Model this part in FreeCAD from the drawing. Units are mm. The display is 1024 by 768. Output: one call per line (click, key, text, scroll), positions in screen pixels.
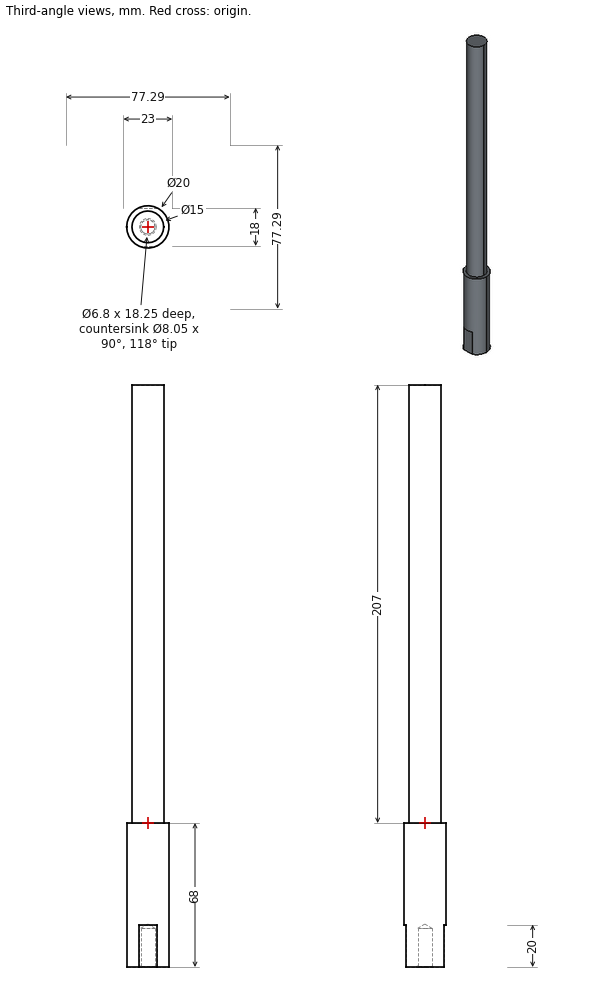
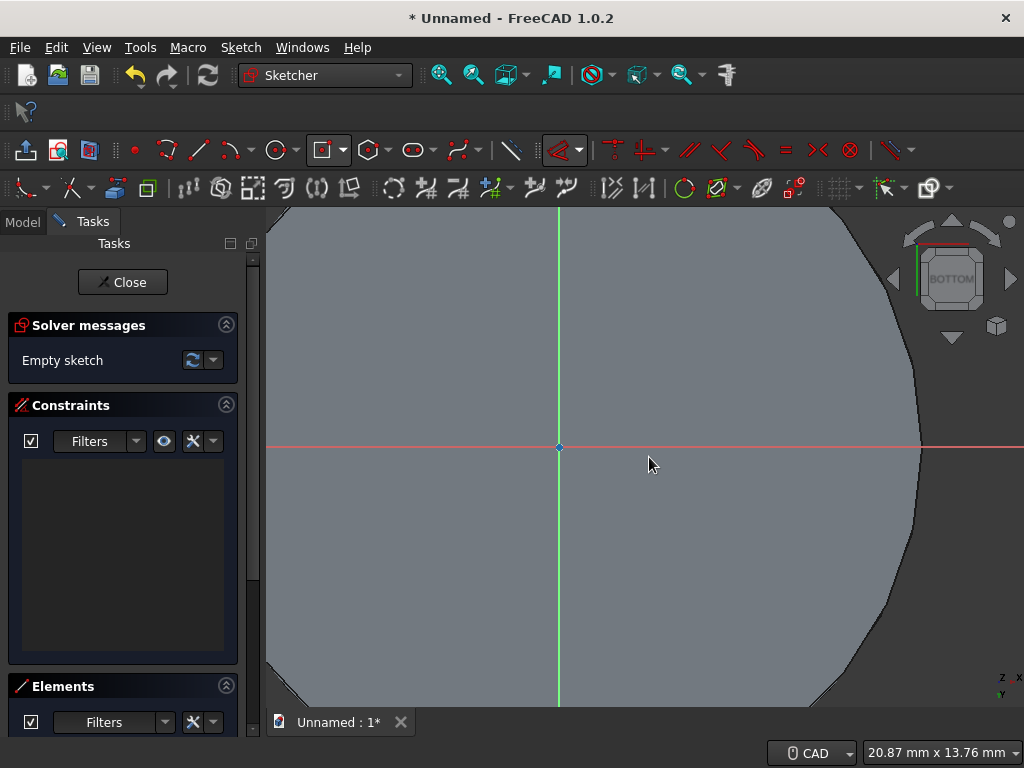
click(276, 150)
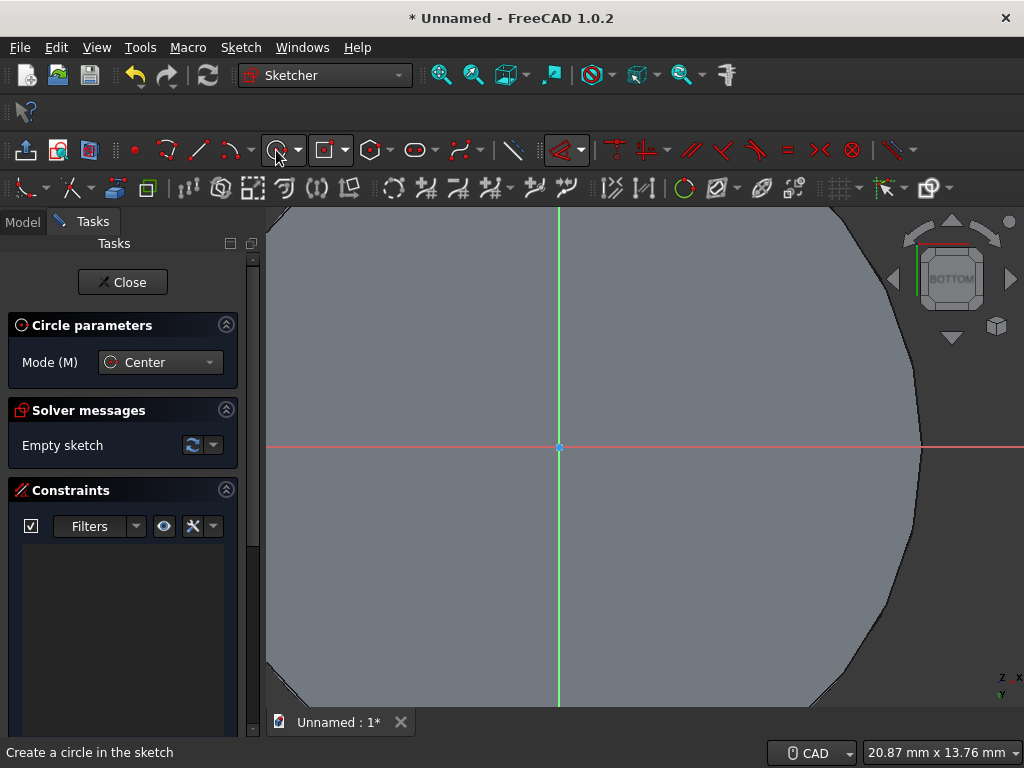
click(559, 447)
click(646, 360)
key(Escape)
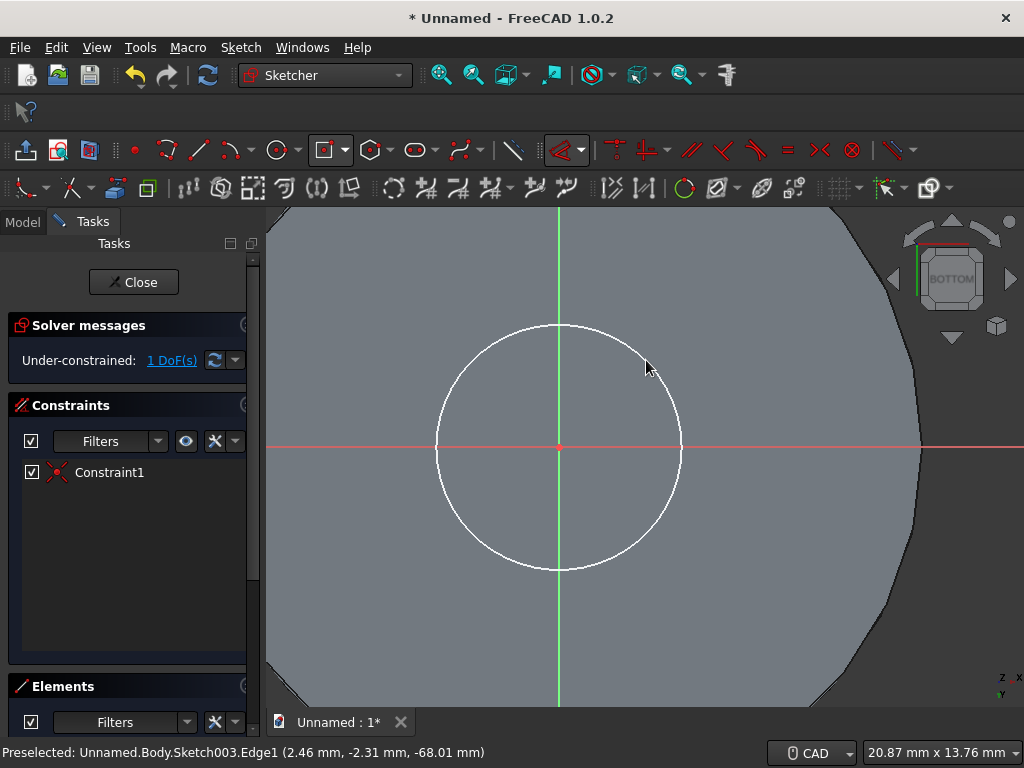
click(645, 360)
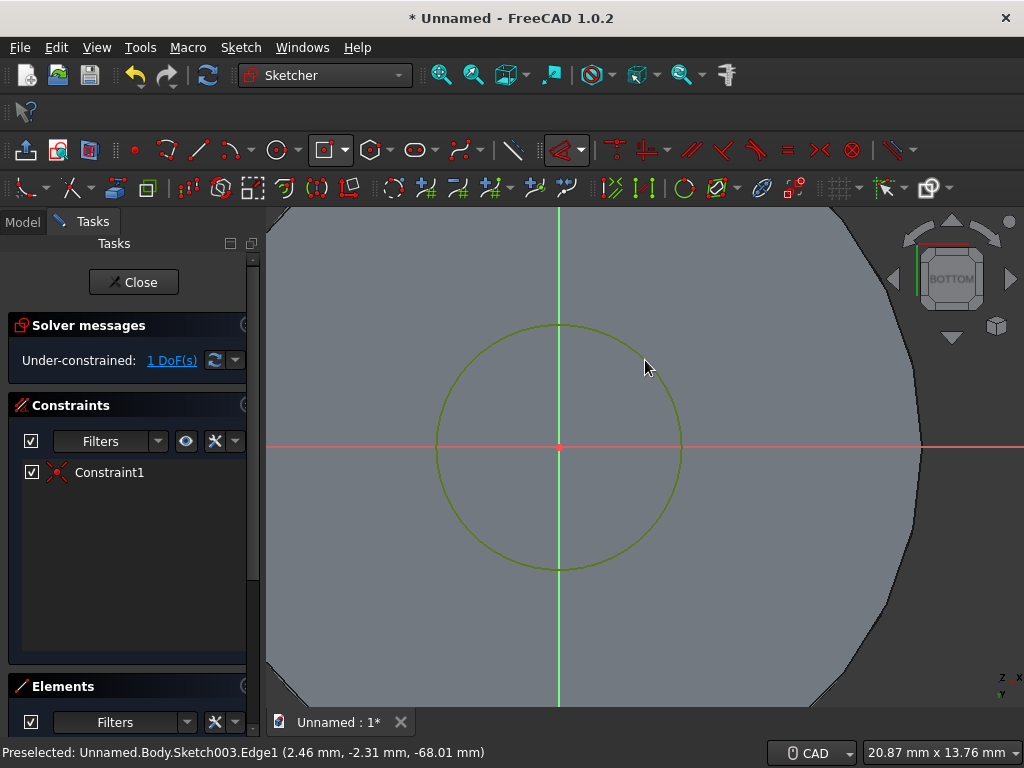
key(k)
key(o)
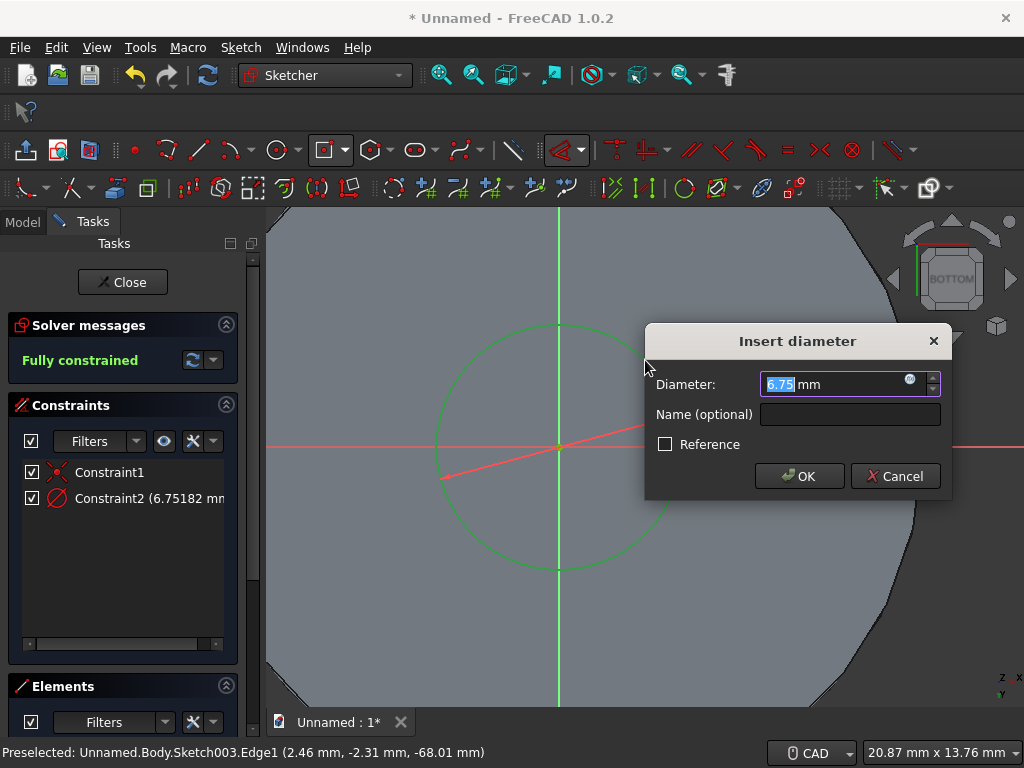
text(6.8)
key(Return)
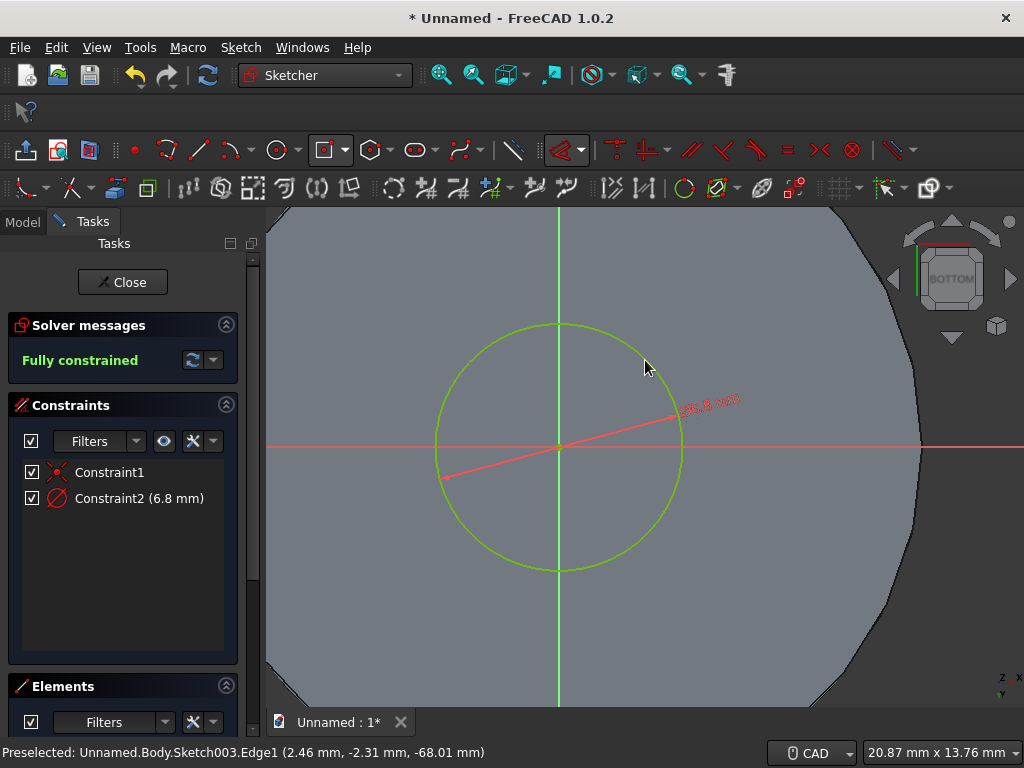
click(123, 282)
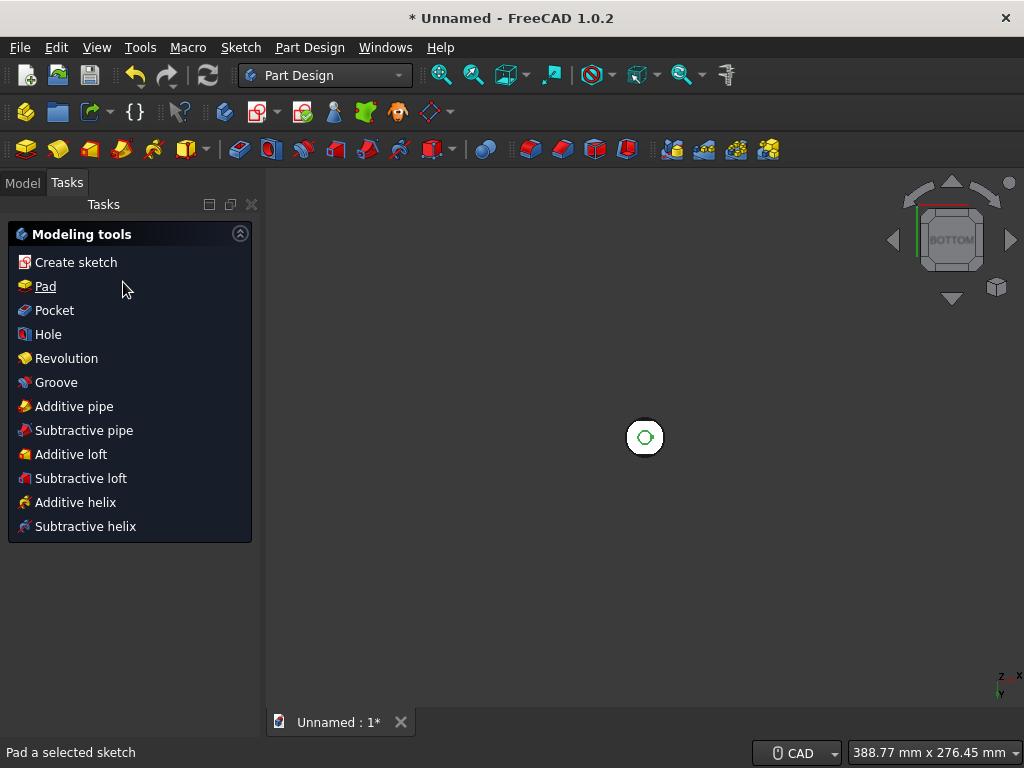
click(272, 150)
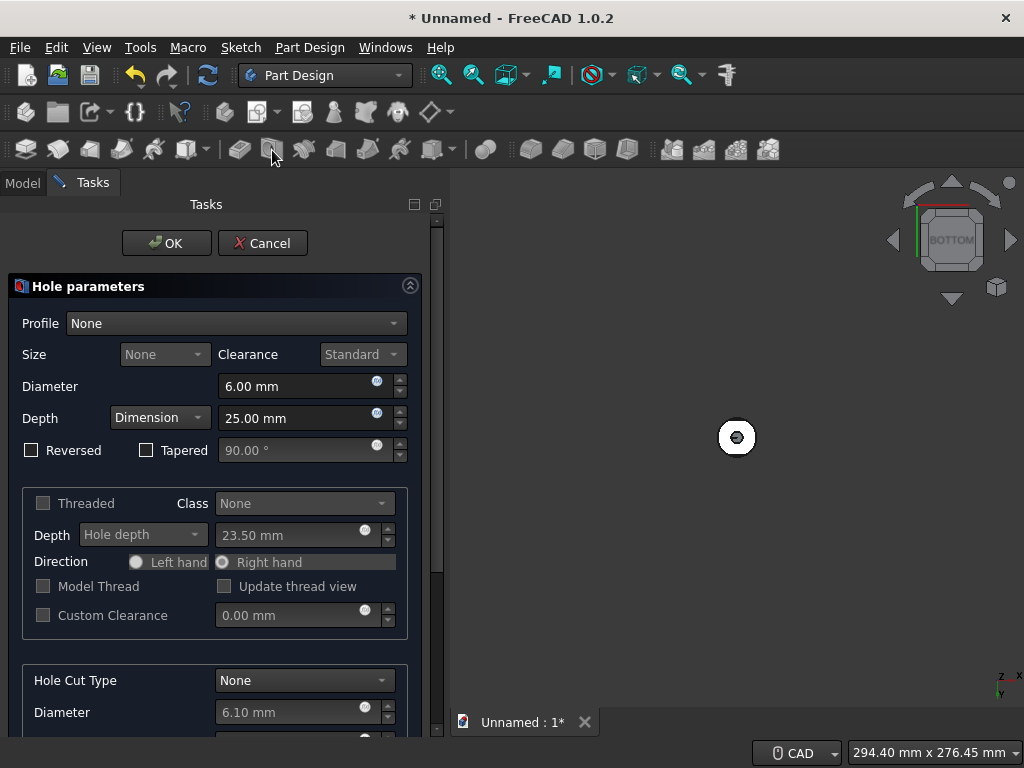
triple_click(305, 386)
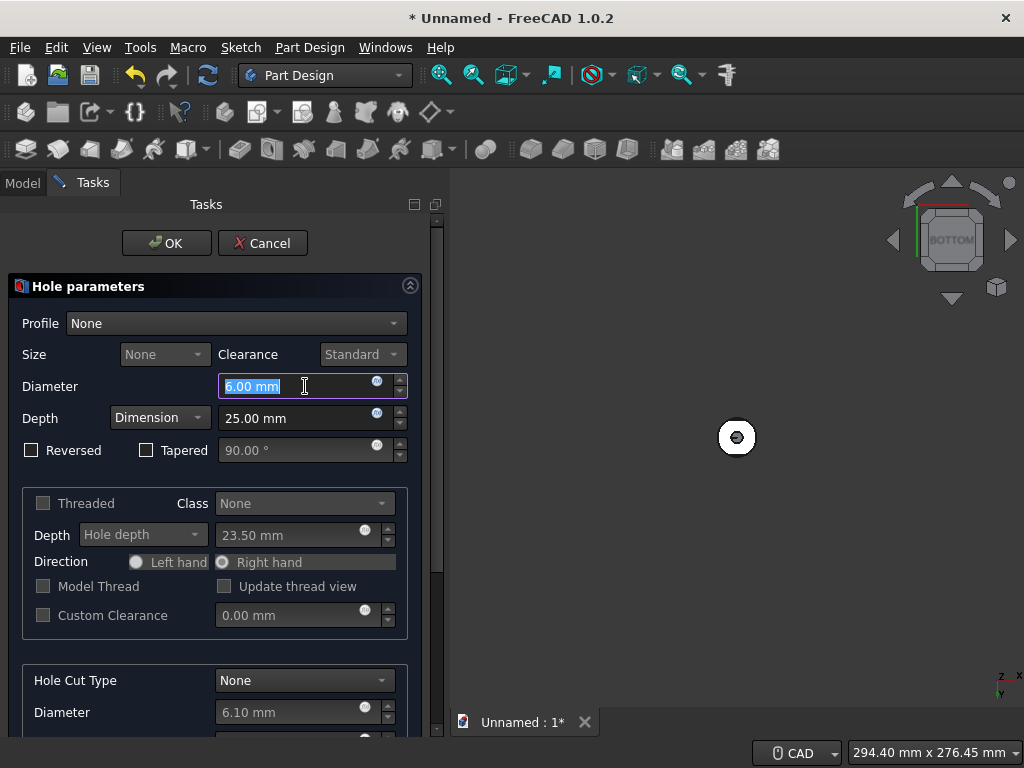
text(6.8)
key(Tab)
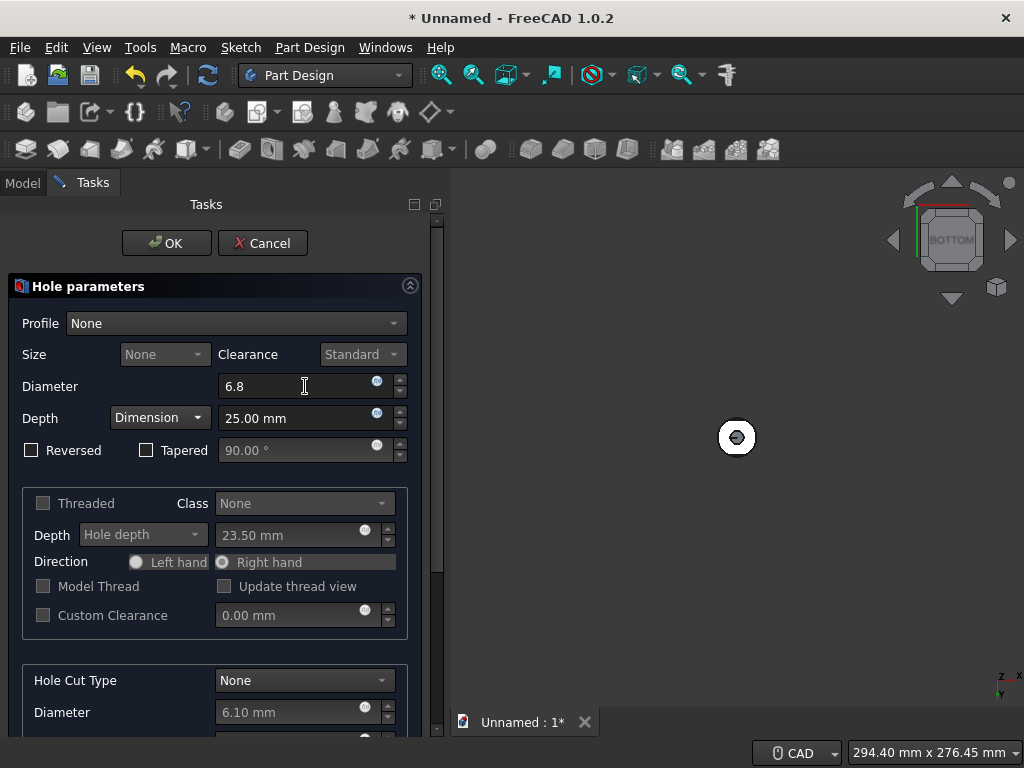
triple_click(305, 418)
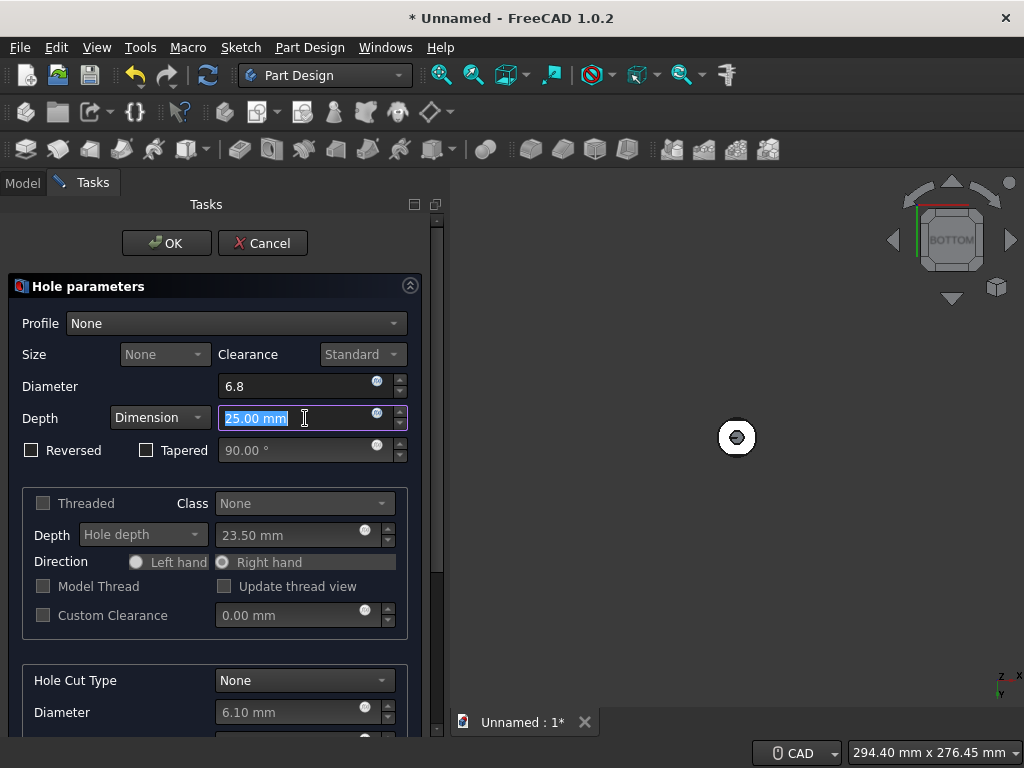
text(18.25)
key(Tab)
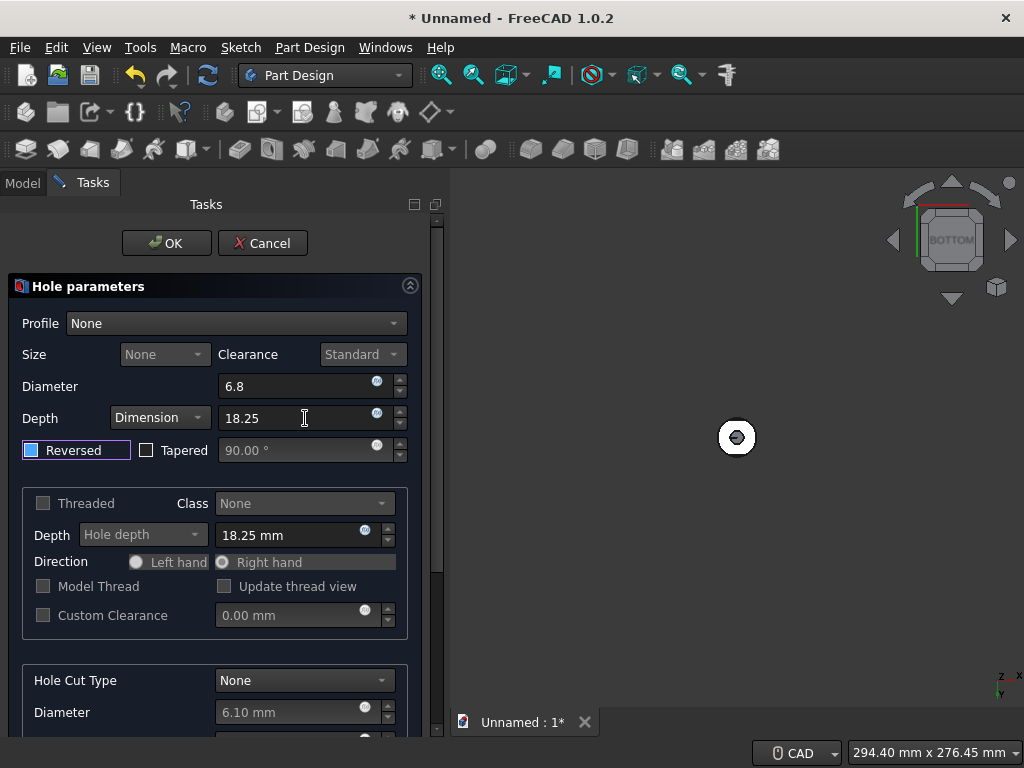
click(306, 680)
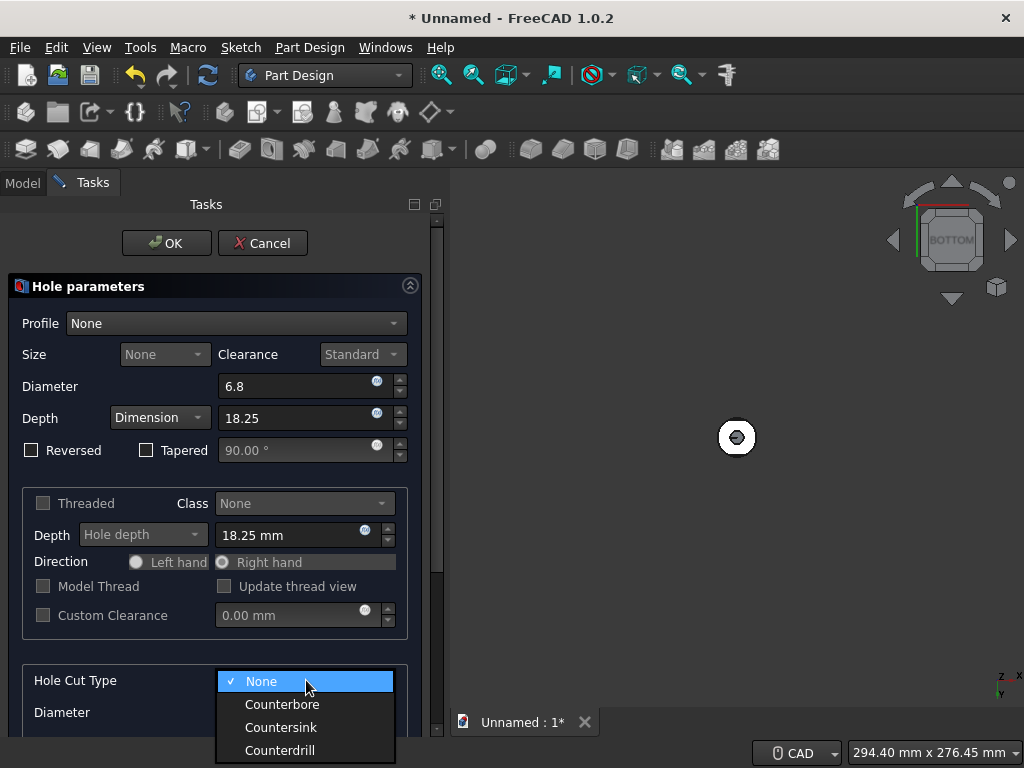
click(304, 728)